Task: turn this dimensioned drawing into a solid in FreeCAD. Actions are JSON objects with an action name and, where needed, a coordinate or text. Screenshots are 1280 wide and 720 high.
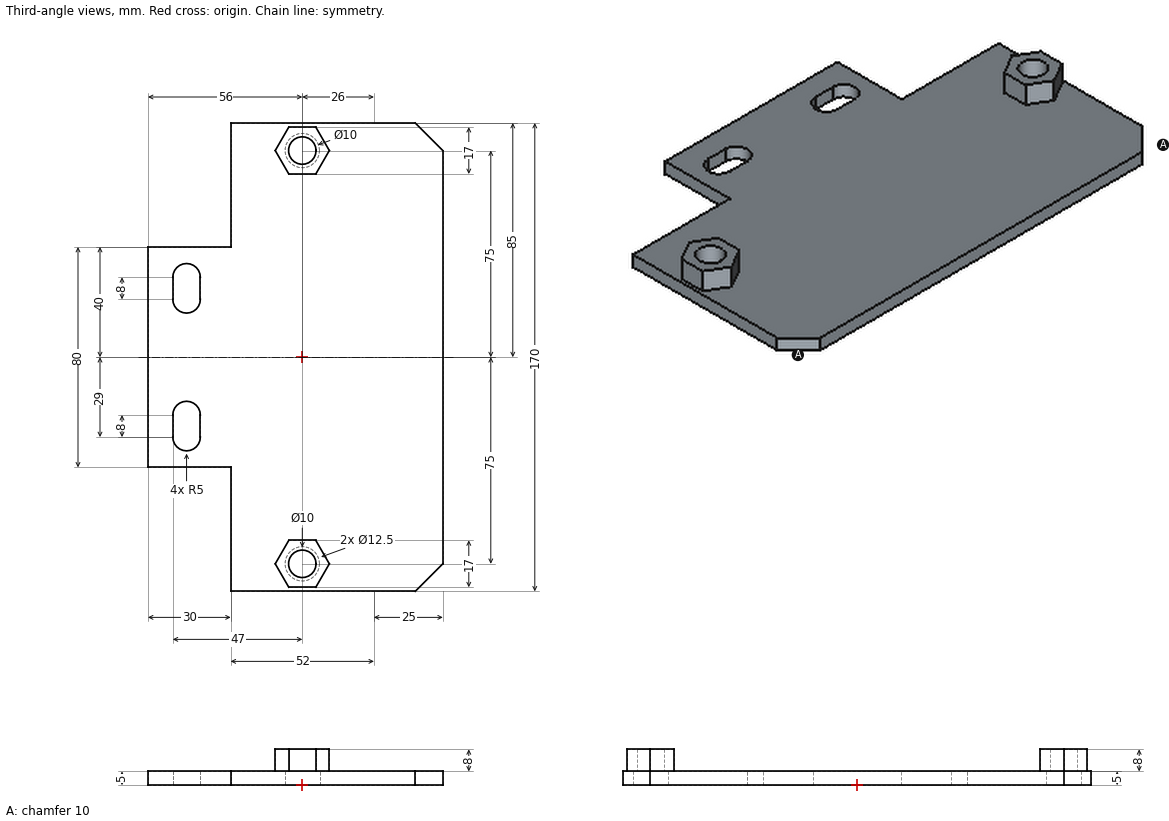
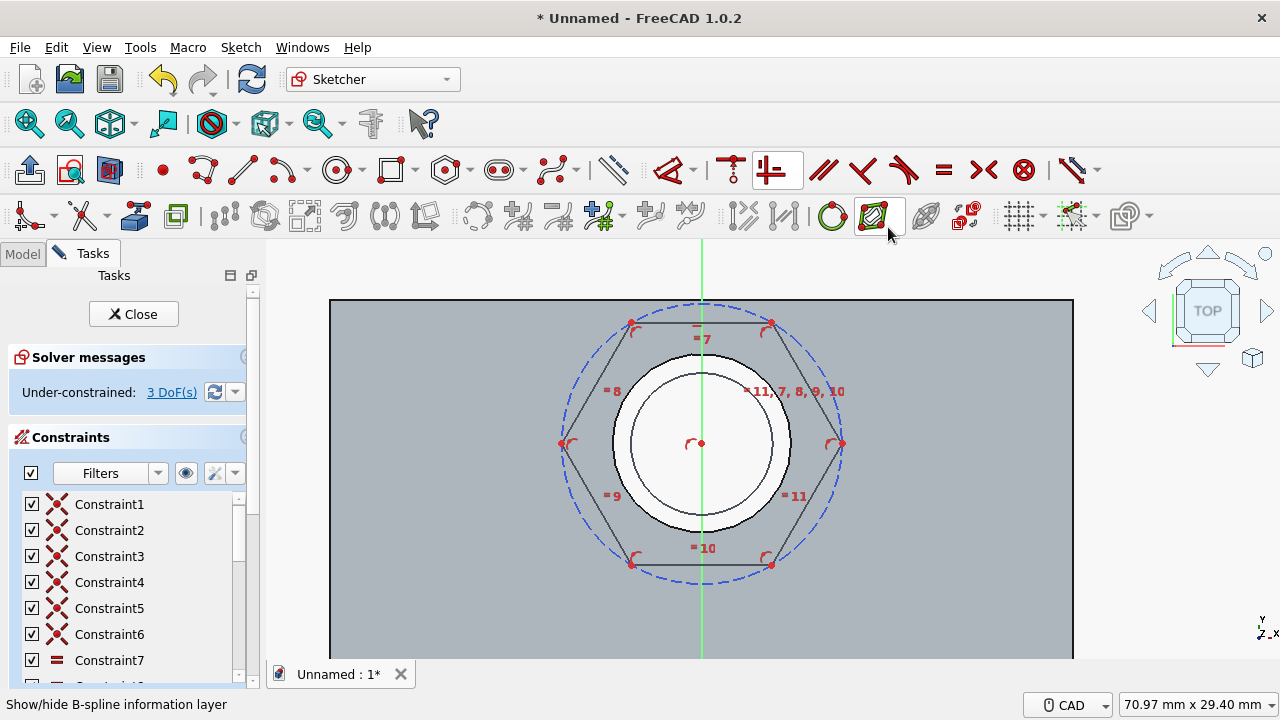
{"action": "left_click", "coordinate": [668, 170]}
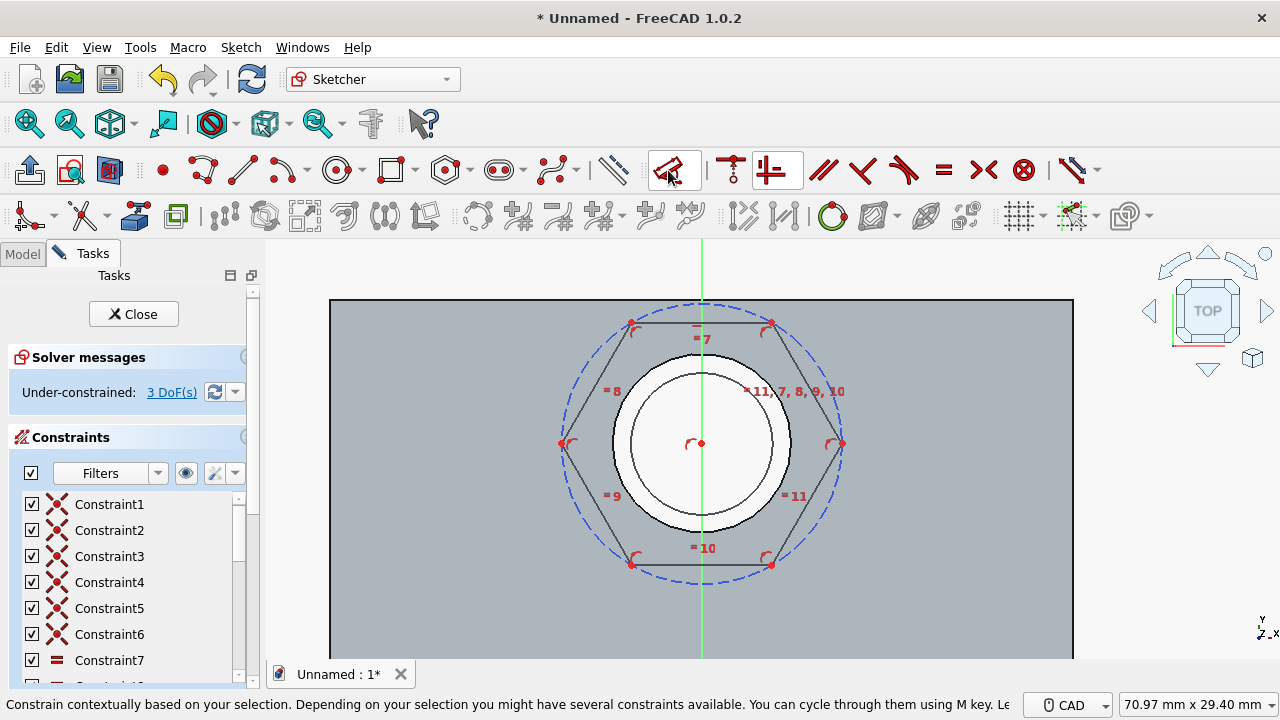
{"action": "left_click", "coordinate": [752, 394]}
{"action": "left_click", "coordinate": [775, 371]}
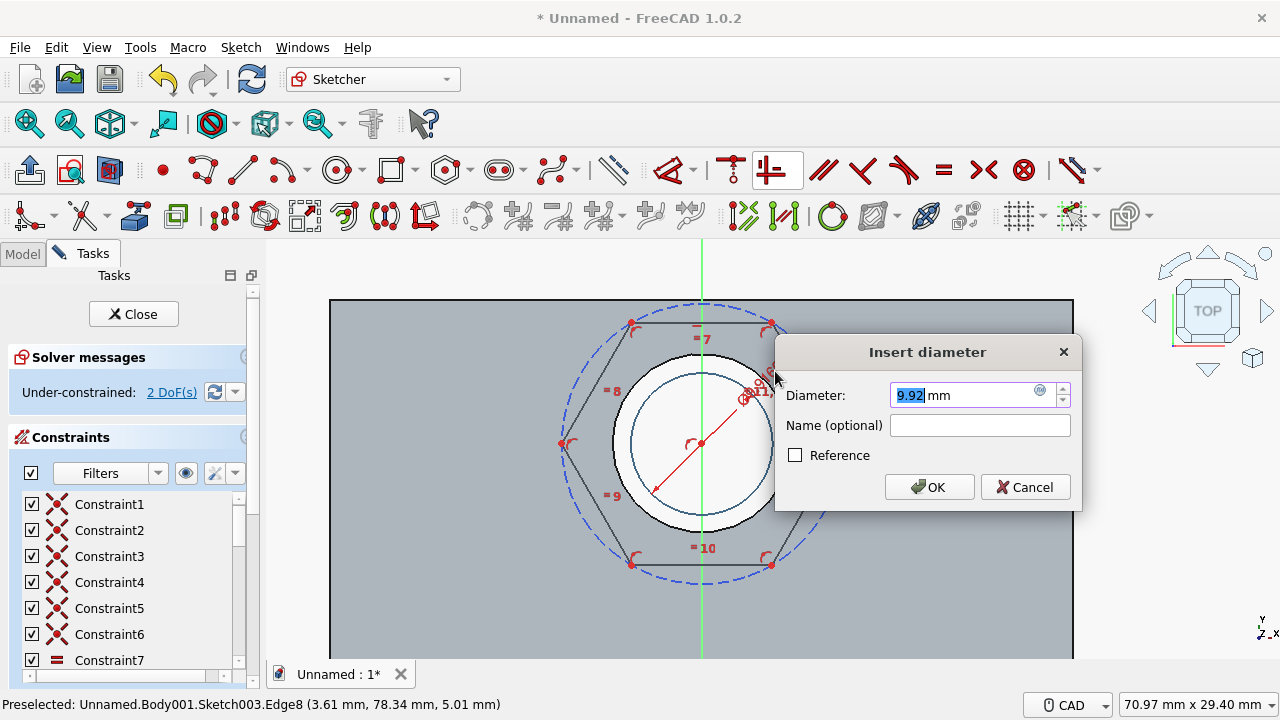
{"action": "type", "text": "10"}
{"action": "key", "text": "Return"}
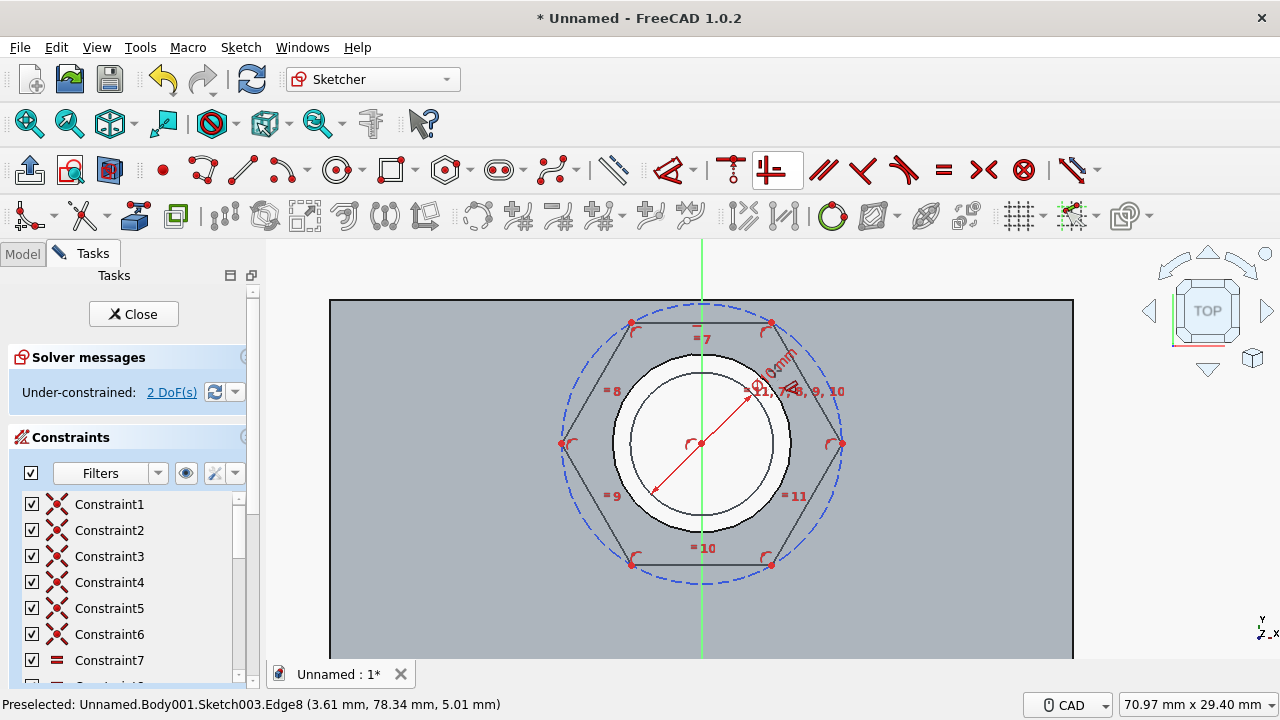
{"action": "left_click", "coordinate": [632, 565]}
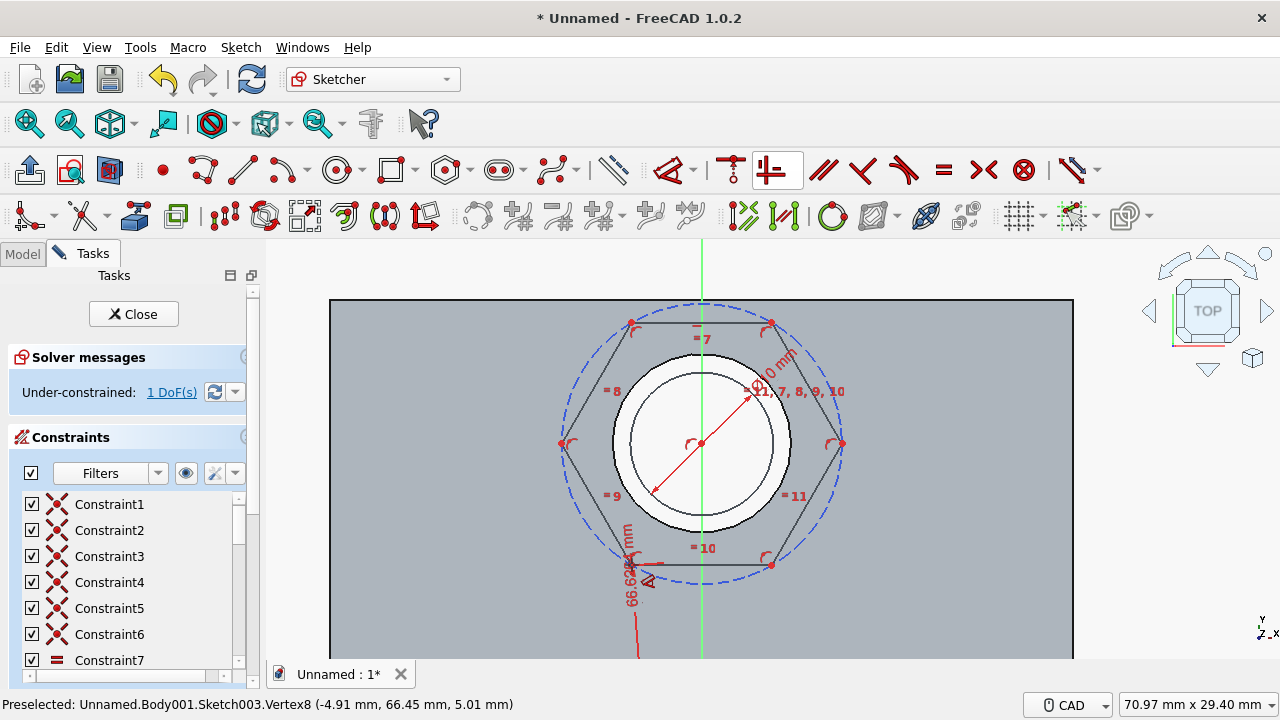
{"action": "left_click", "coordinate": [772, 323]}
{"action": "left_click", "coordinate": [598, 444]}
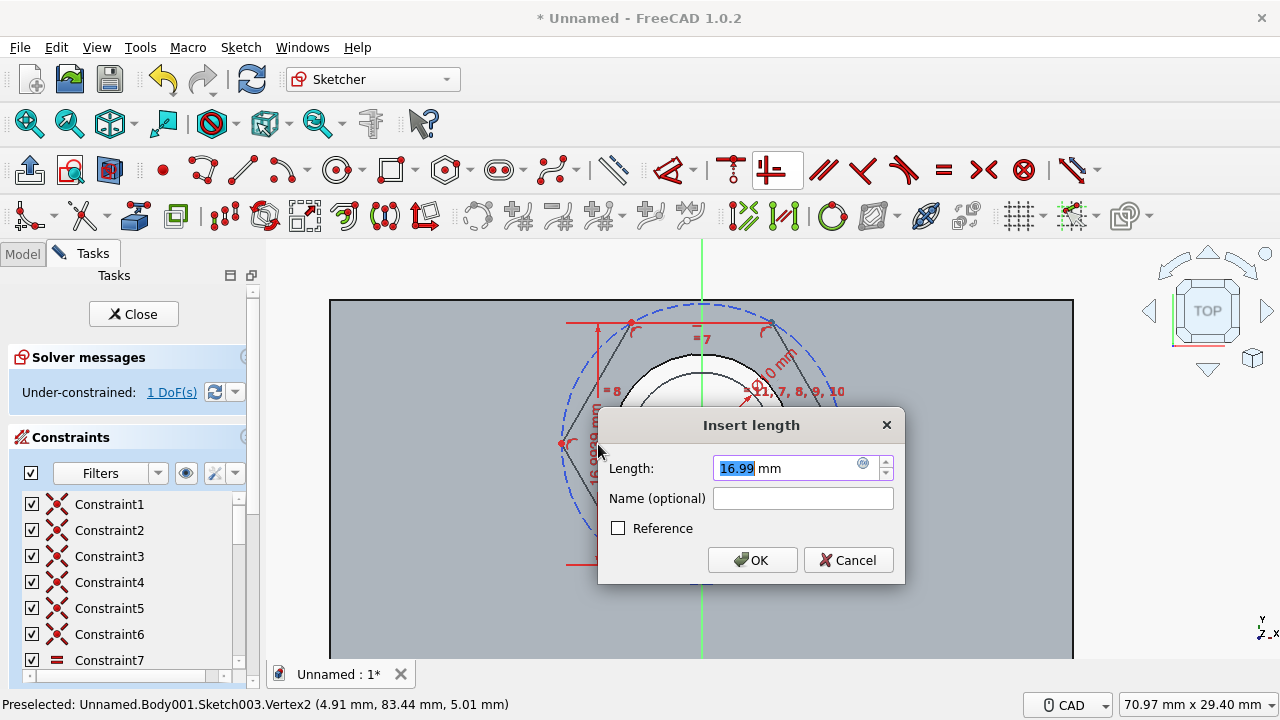
{"action": "type", "text": "17"}
{"action": "key", "text": "Return"}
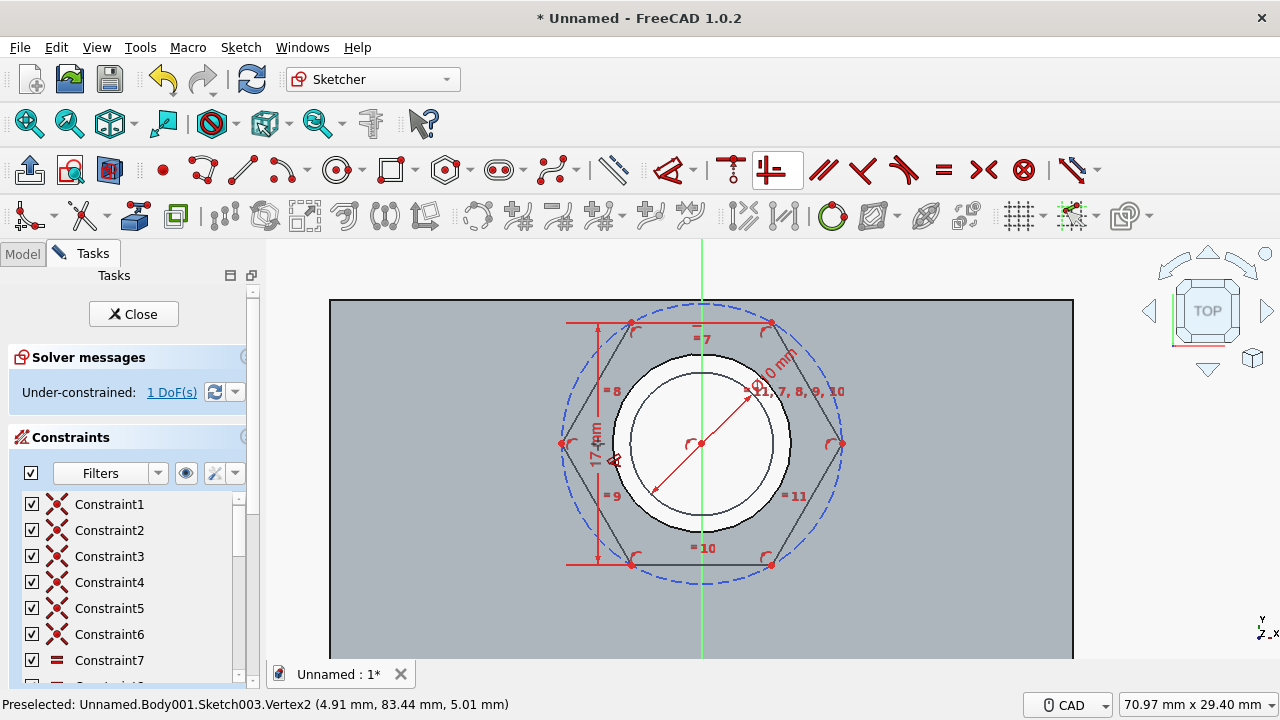
{"action": "left_click", "coordinate": [702, 444]}
{"action": "left_click", "coordinate": [736, 537]}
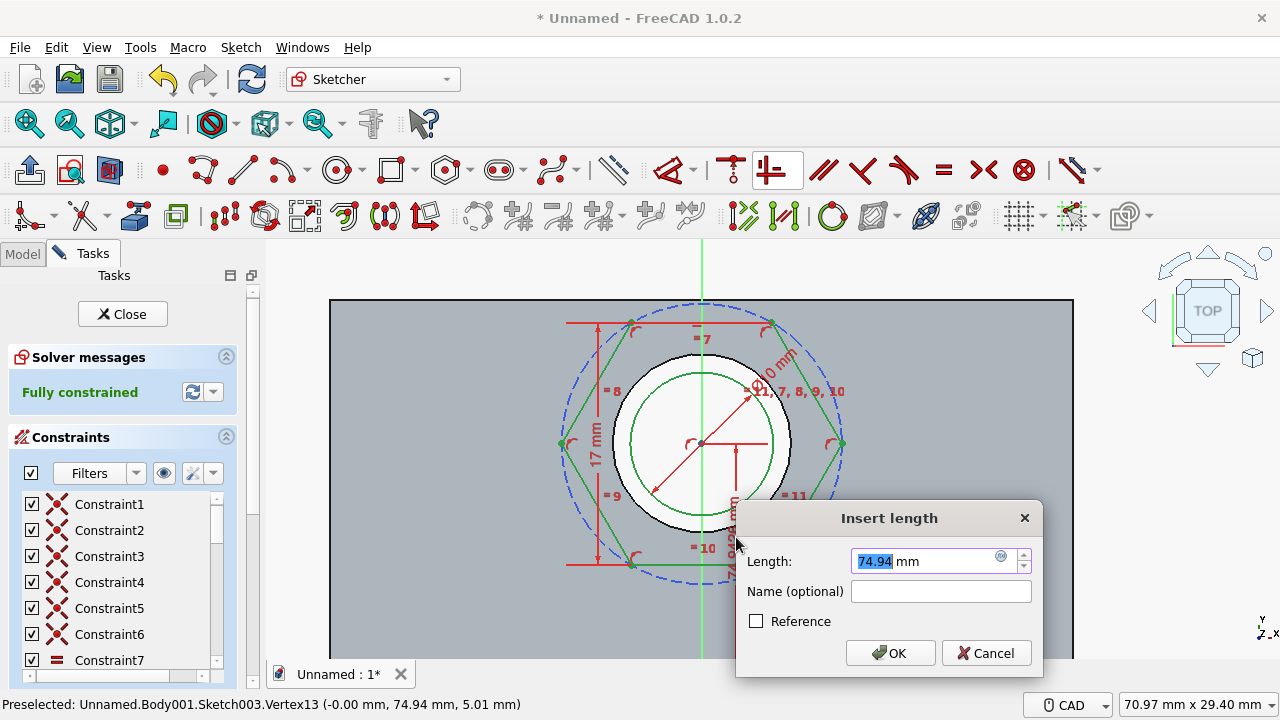
{"action": "type", "text": "75"}
{"action": "key", "text": "Return"}
{"action": "key", "text": "Escape"}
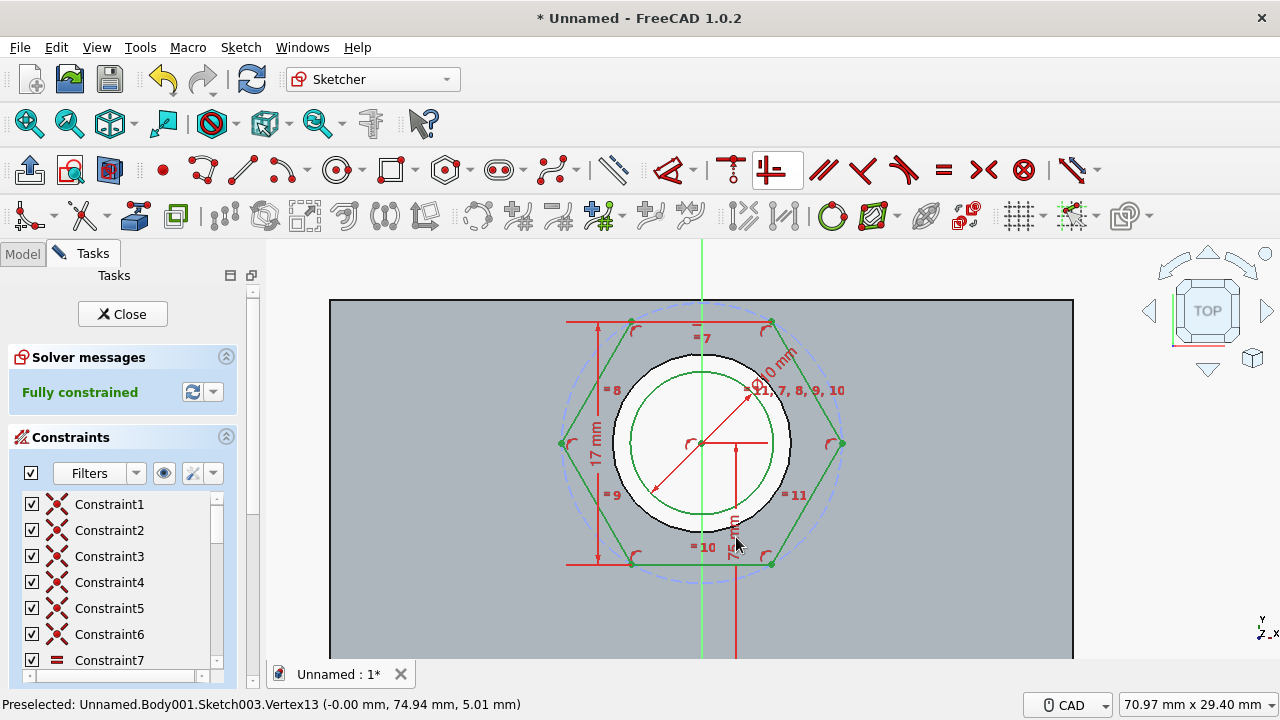
{"action": "left_click", "coordinate": [123, 314]}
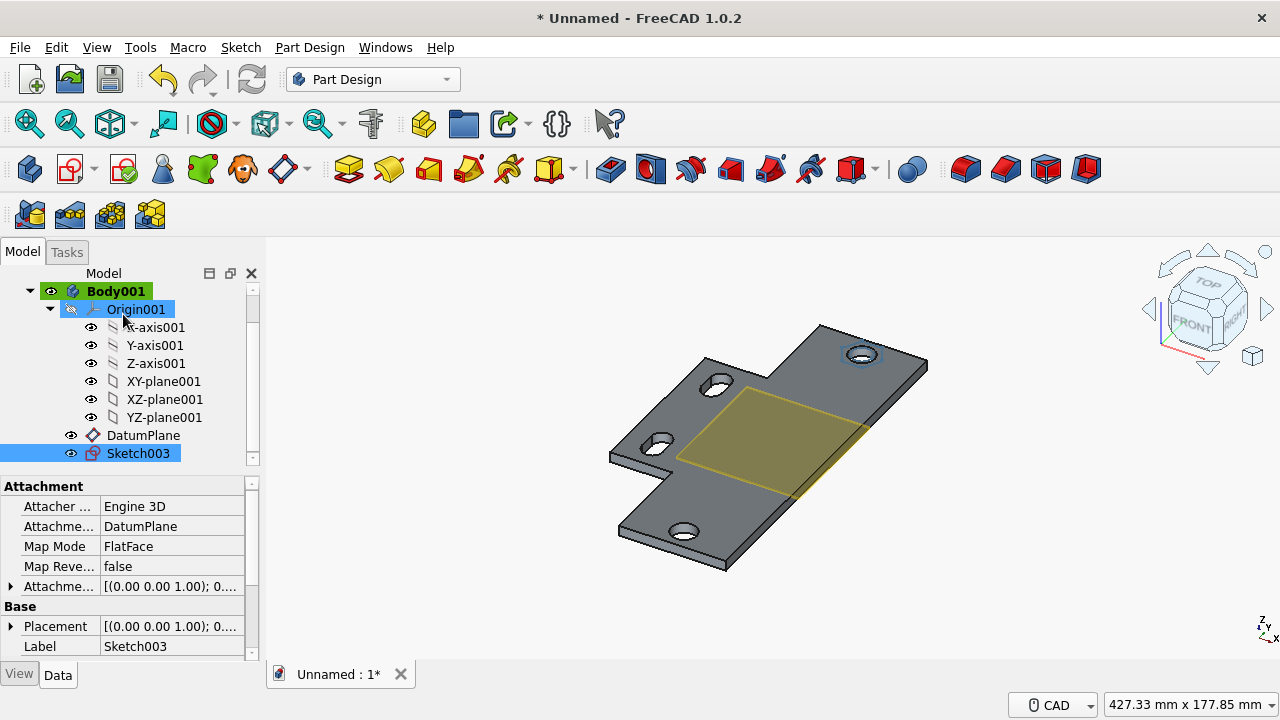
{"action": "left_click", "coordinate": [350, 170]}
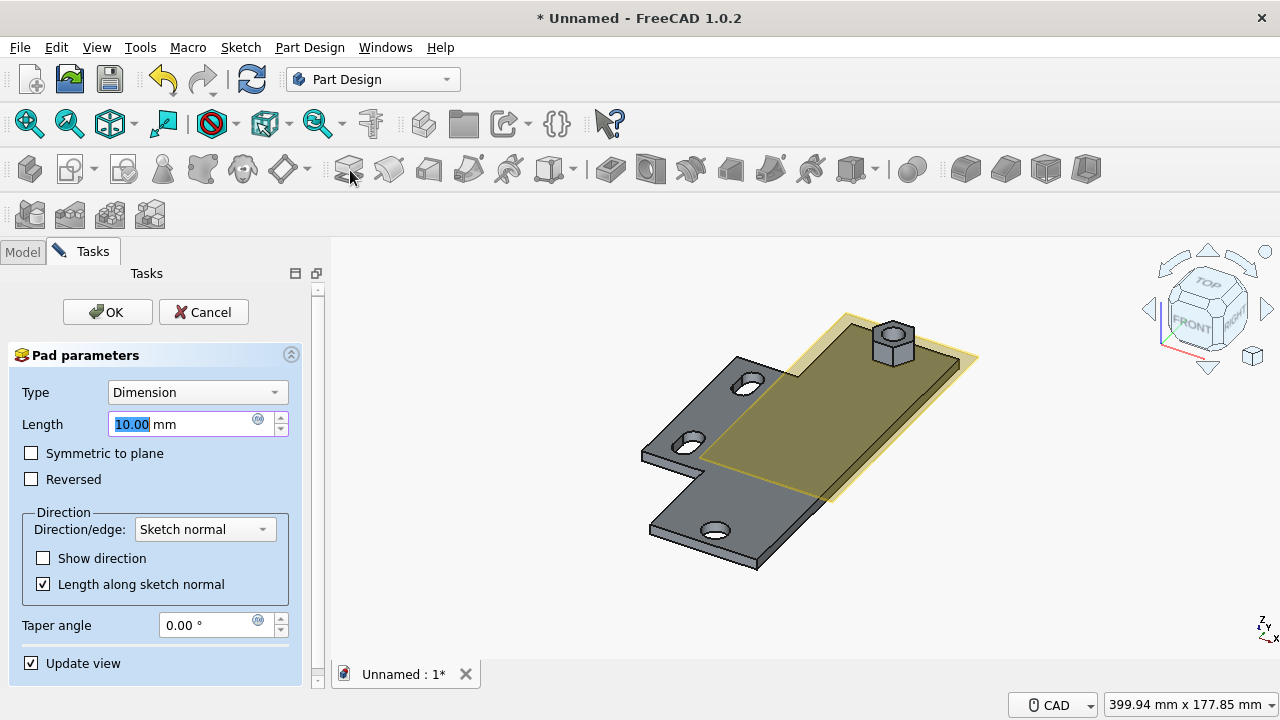
{"action": "type", "text": "8"}
{"action": "key", "text": "Tab"}